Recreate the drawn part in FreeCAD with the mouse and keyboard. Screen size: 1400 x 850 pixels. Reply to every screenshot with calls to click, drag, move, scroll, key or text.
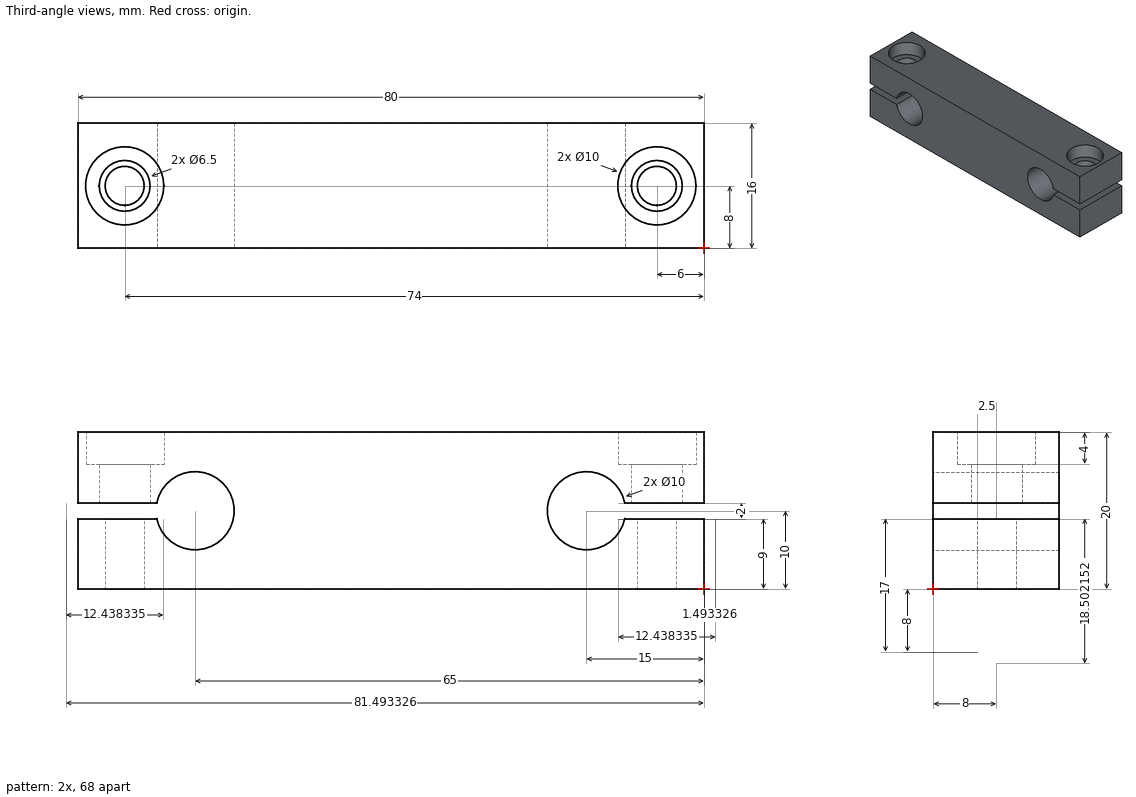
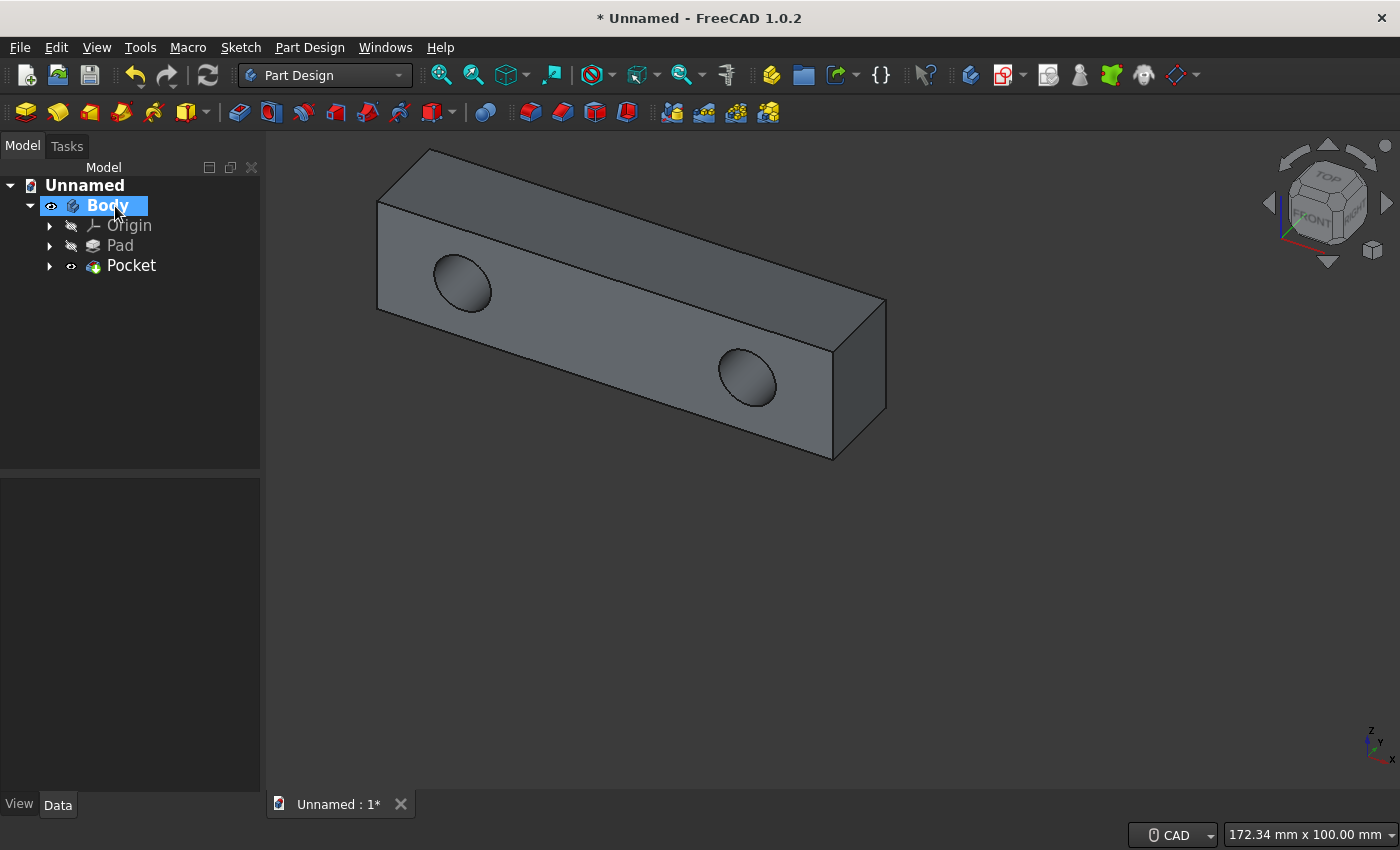
click(605, 330)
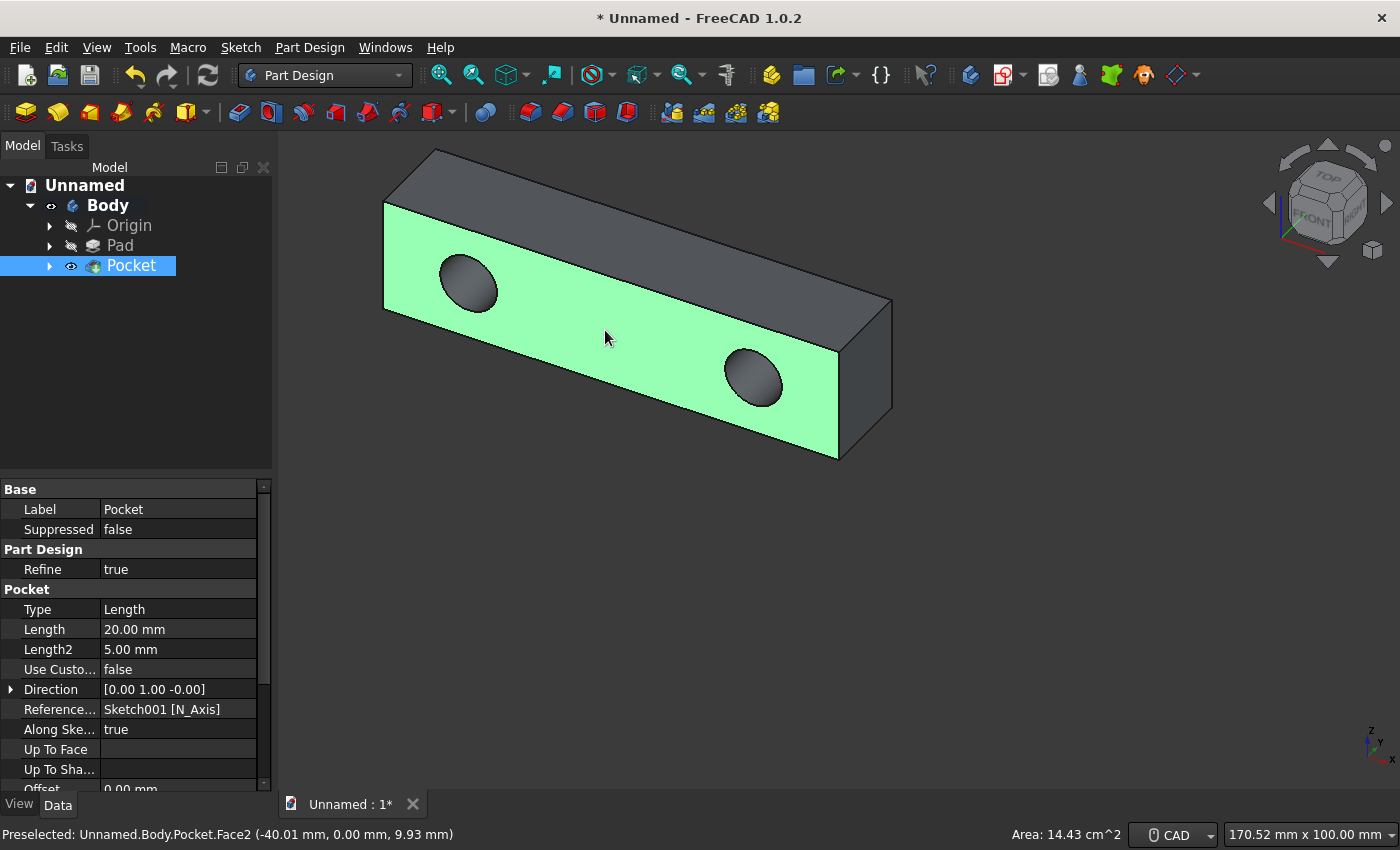
click(1004, 76)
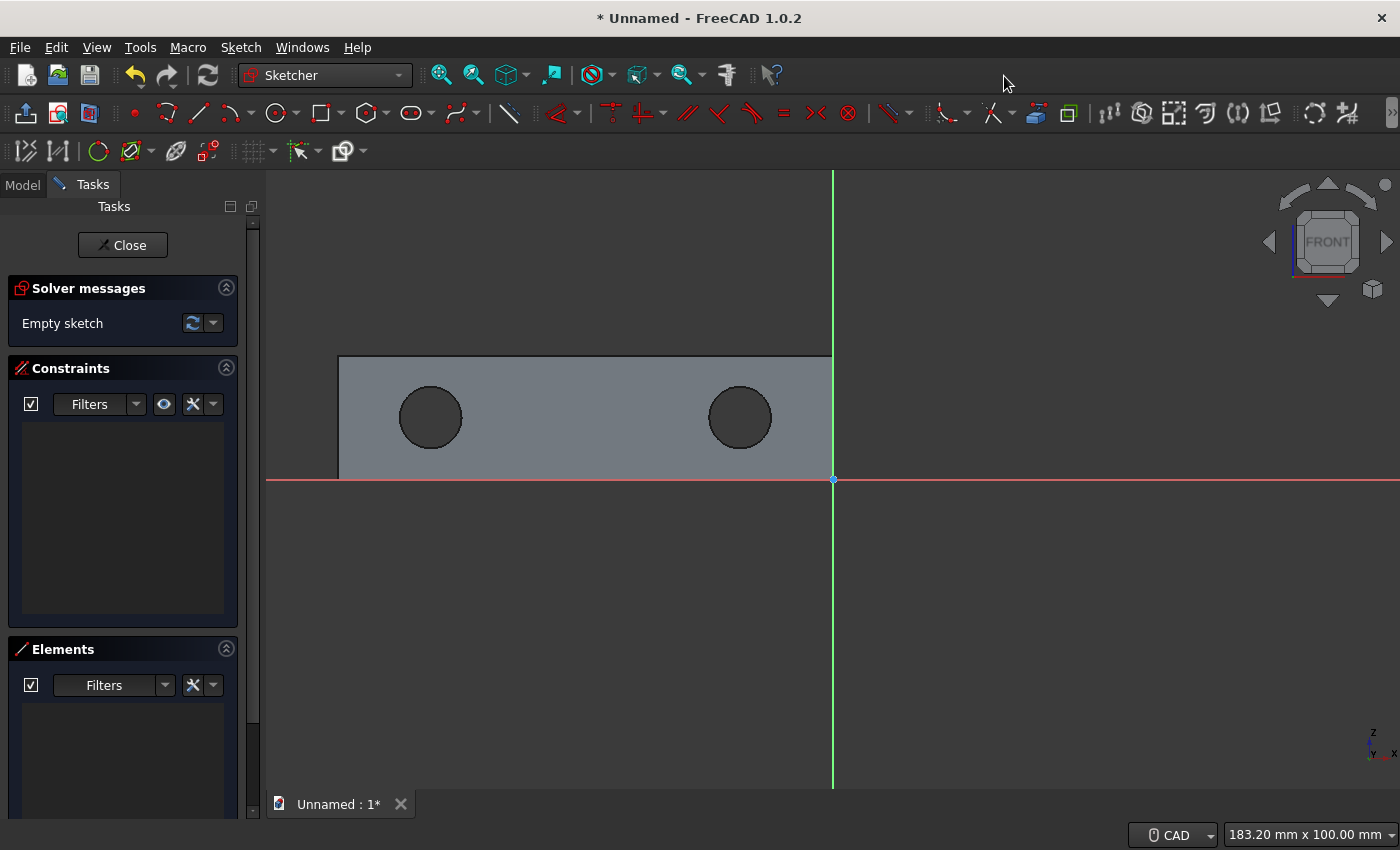
click(322, 114)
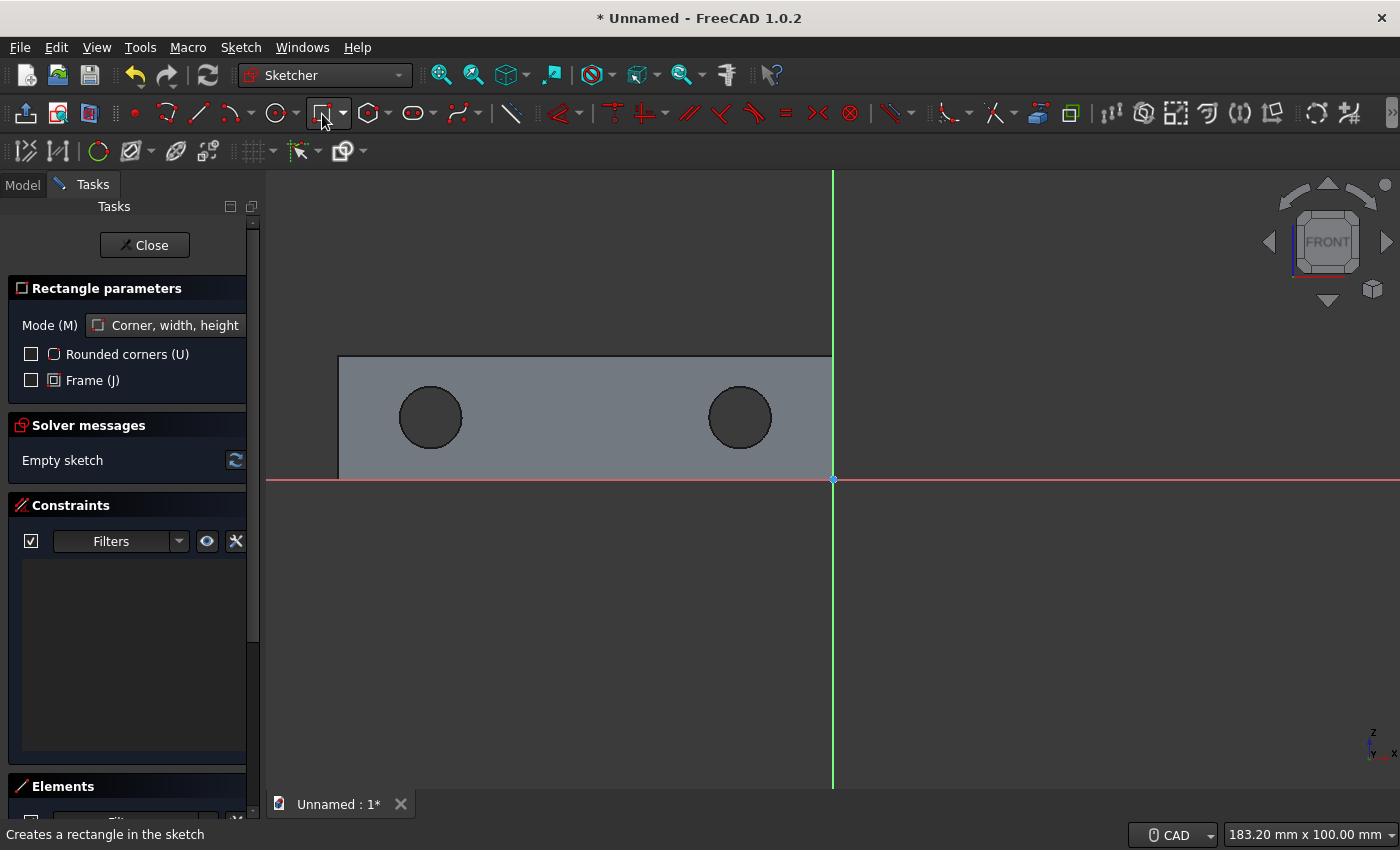
scroll(765, 411, up, 2)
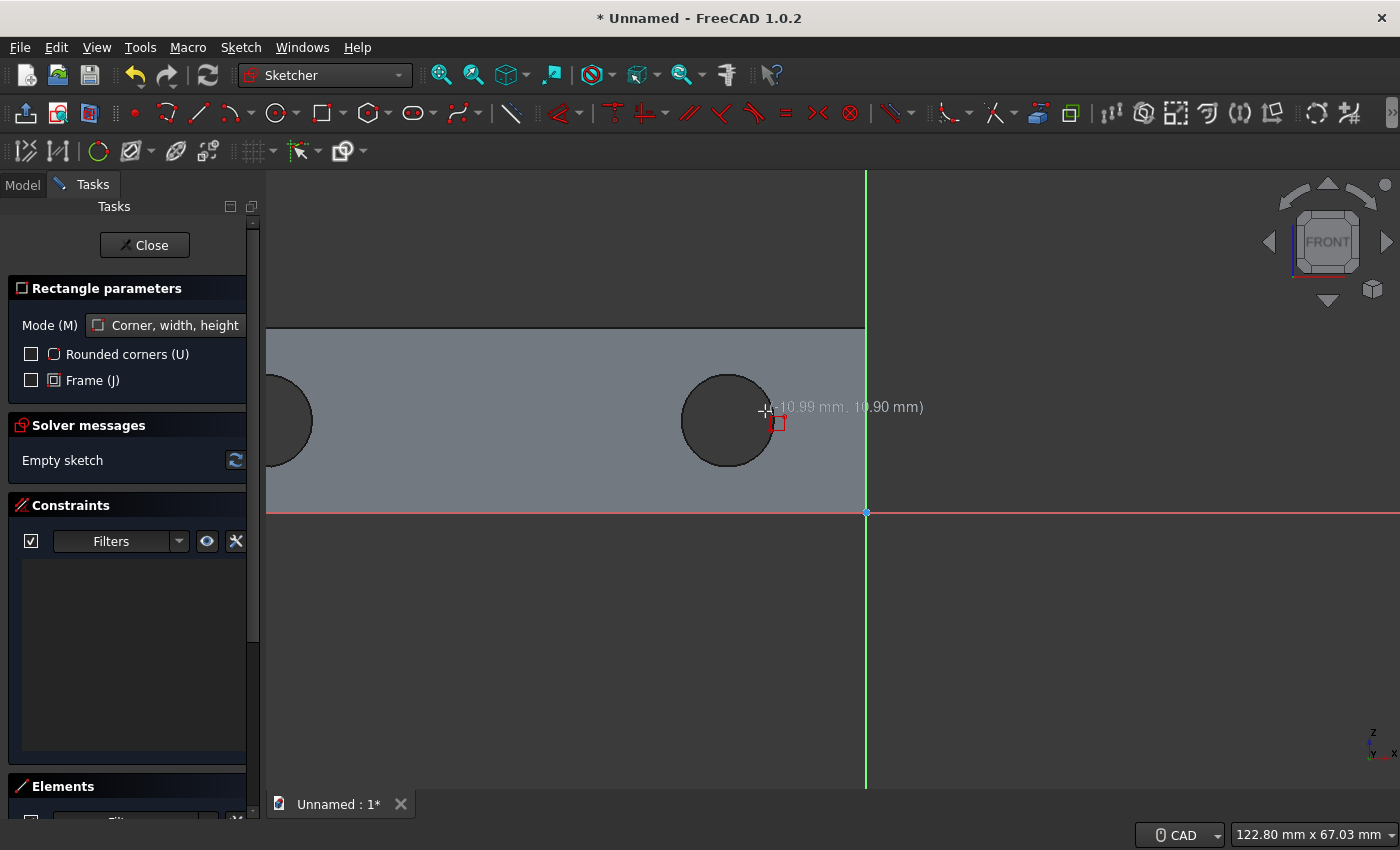
click(765, 411)
click(880, 430)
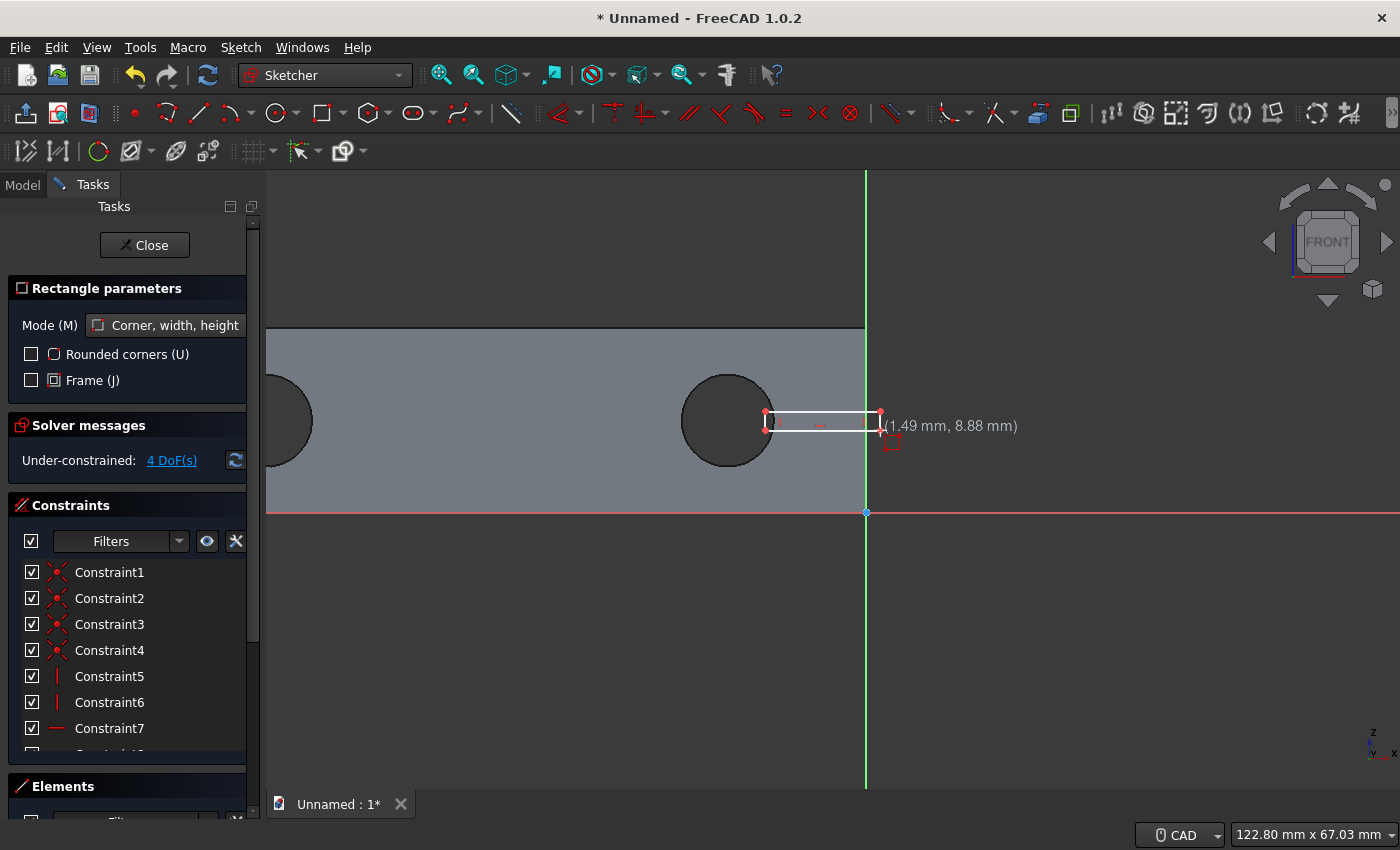
scroll(1235, 515, down, 2)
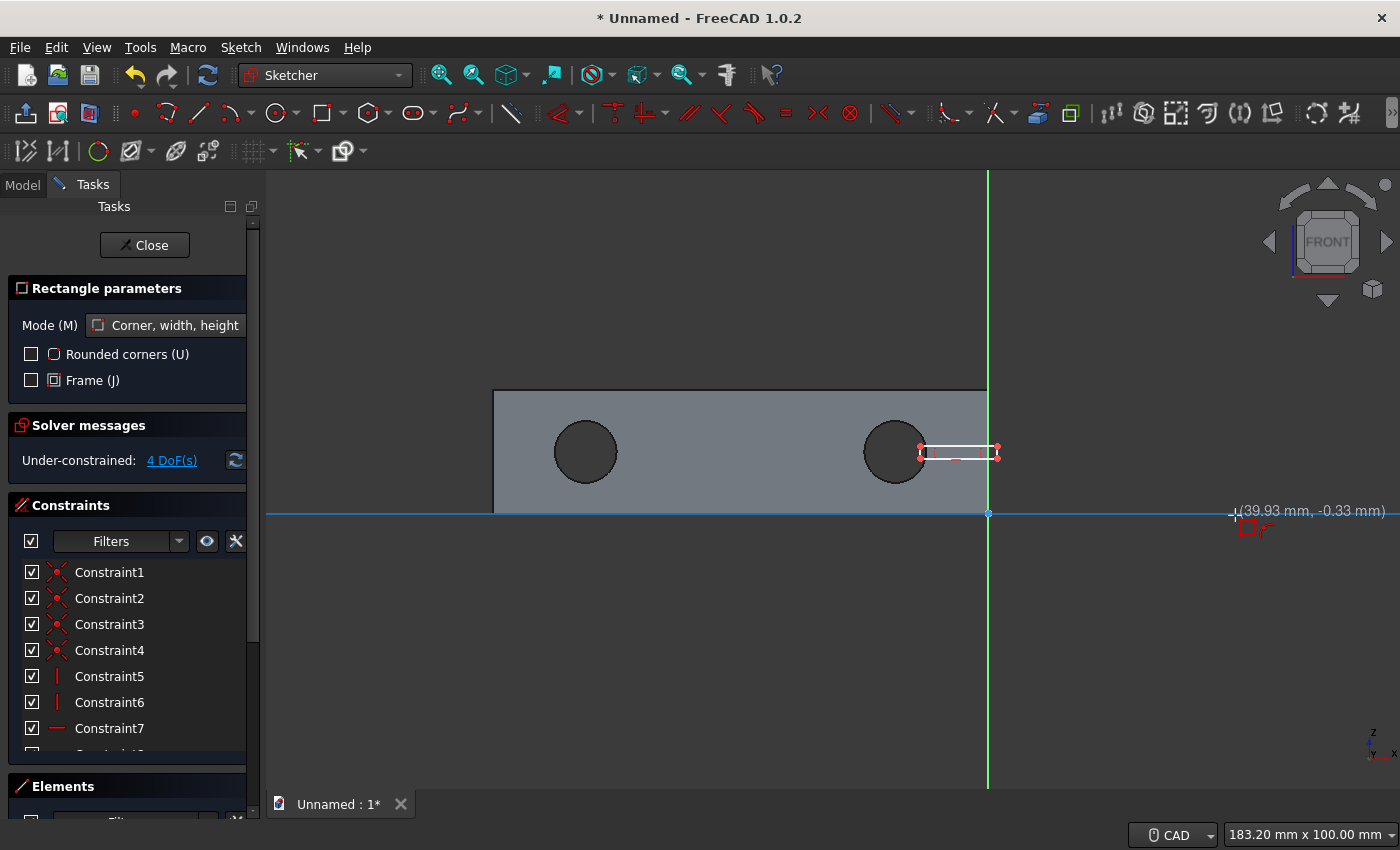
scroll(484, 446, up, 2)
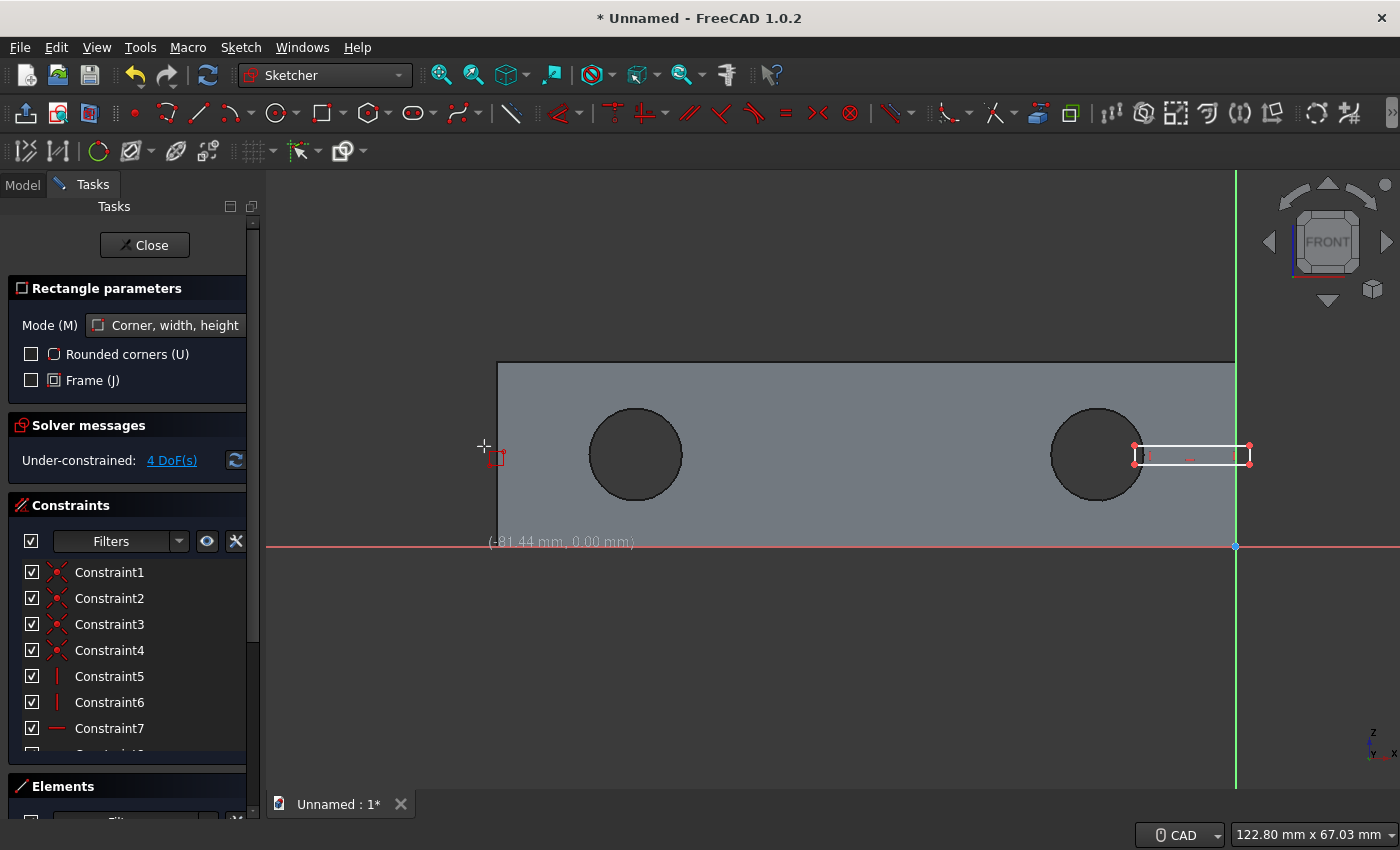
click(483, 445)
click(598, 464)
key(Escape)